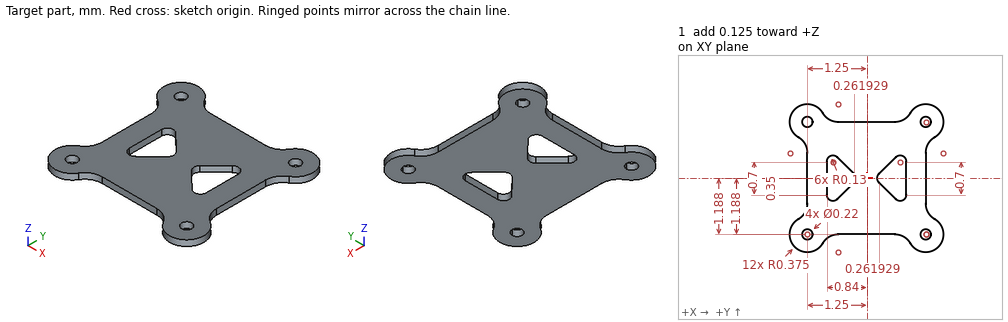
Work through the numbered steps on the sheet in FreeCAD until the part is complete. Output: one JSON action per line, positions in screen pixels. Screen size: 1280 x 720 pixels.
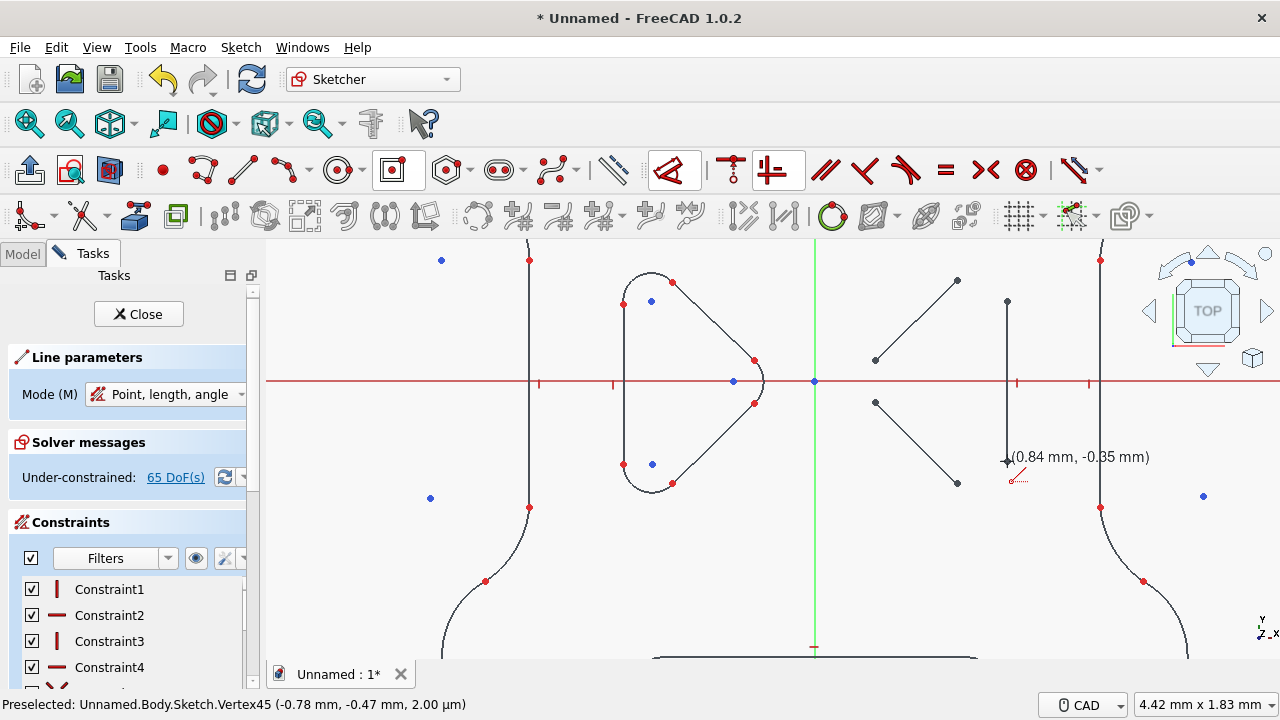
{"action": "left_click", "coordinate": [284, 170]}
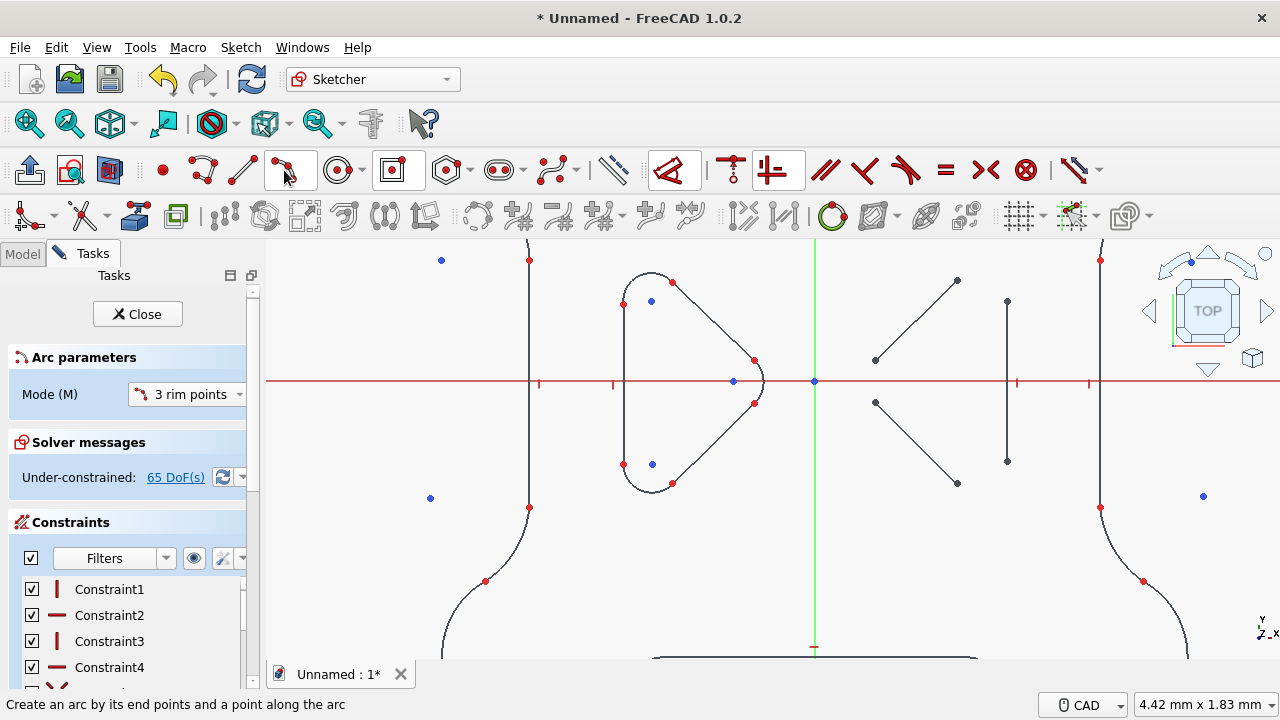
{"action": "left_click", "coordinate": [875, 403]}
{"action": "left_click", "coordinate": [875, 361]}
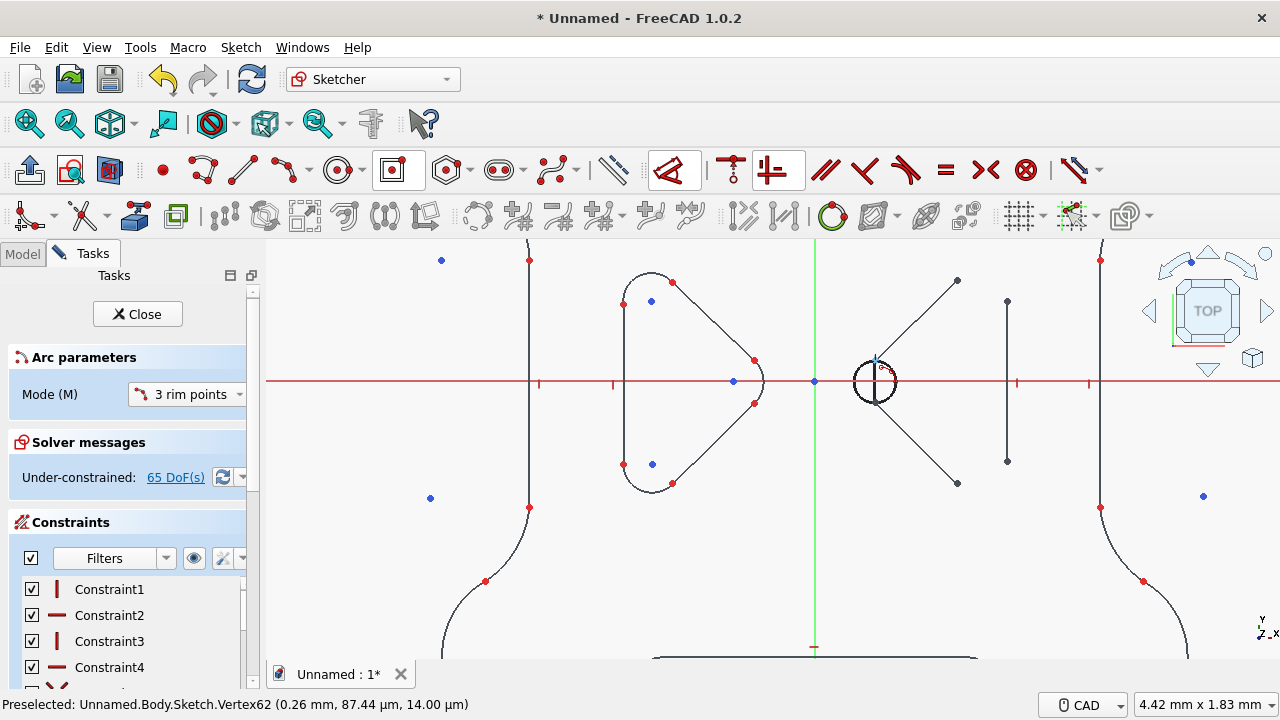
{"action": "scroll", "coordinate": [867, 372], "scroll_direction": "up", "scroll_amount": 4}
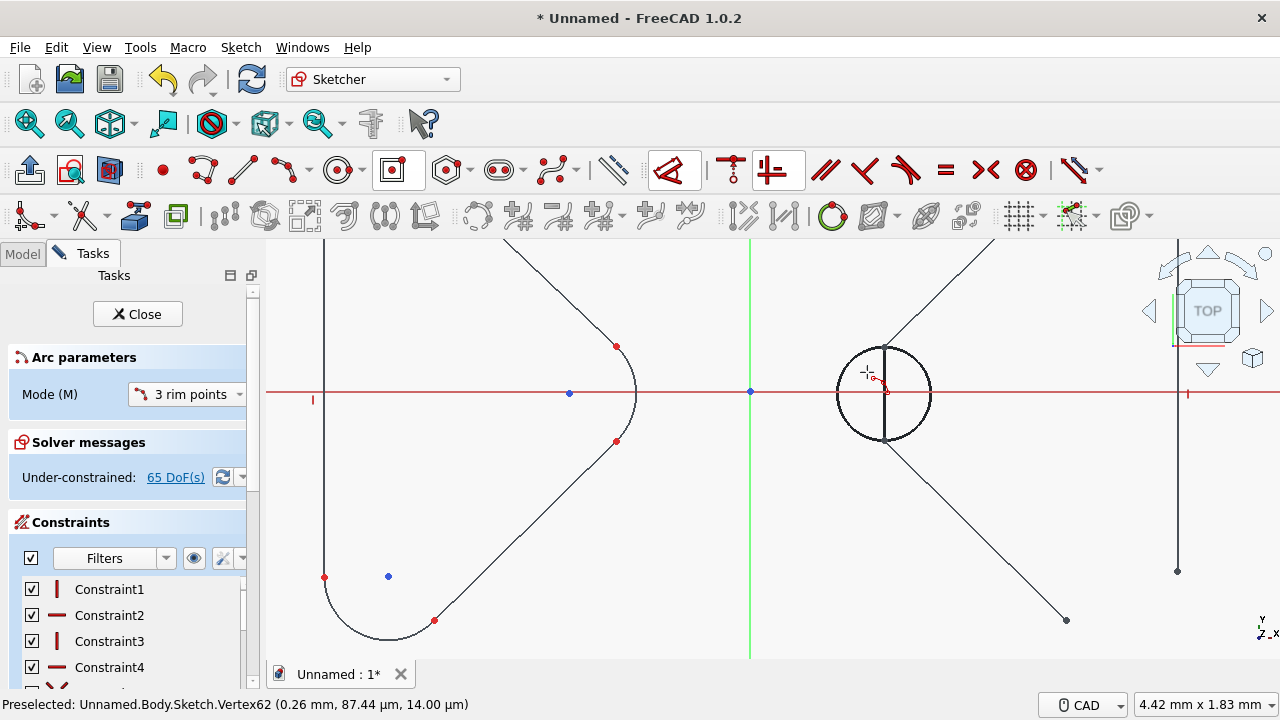
{"action": "left_click", "coordinate": [867, 371]}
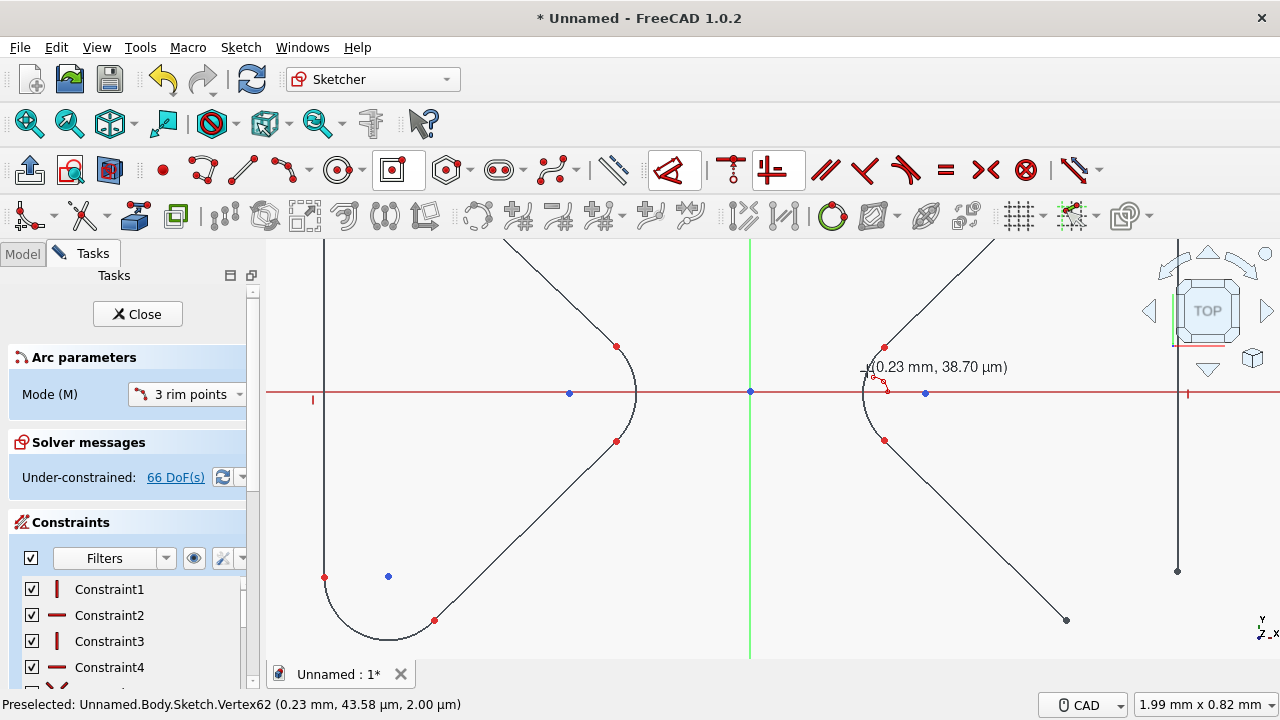
{"action": "scroll", "coordinate": [695, 460], "scroll_direction": "down", "scroll_amount": 9}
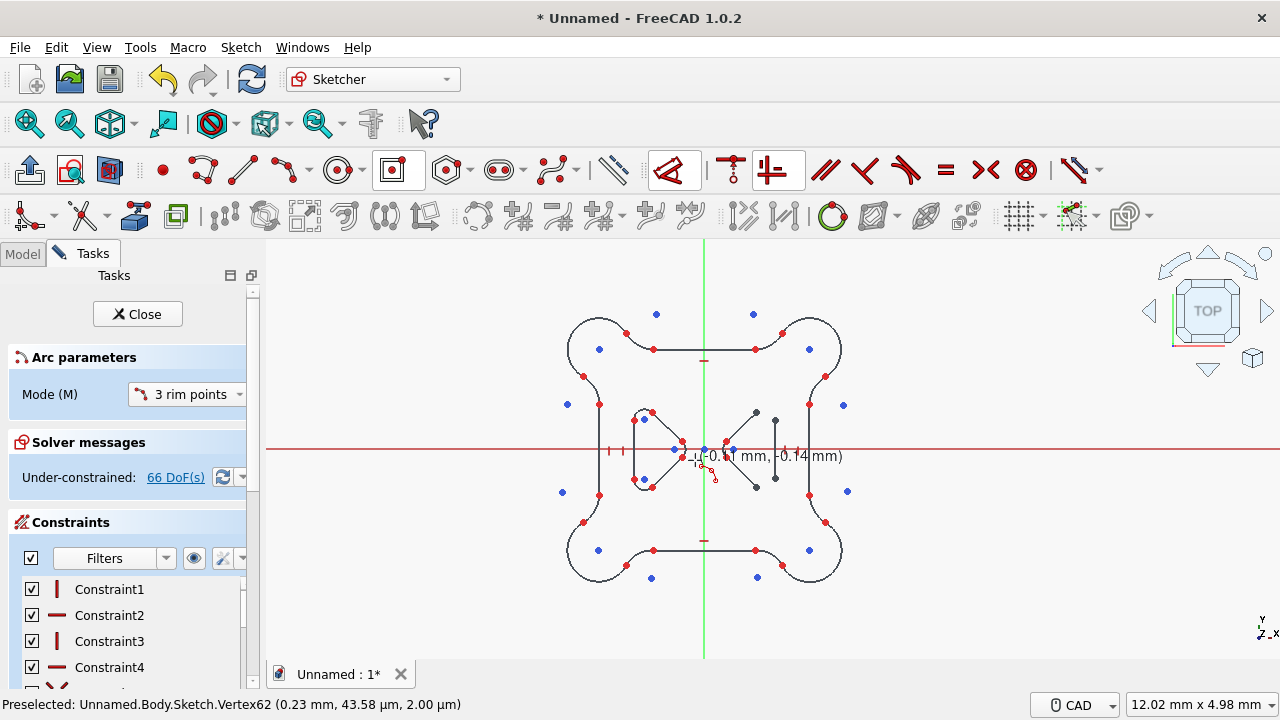
{"action": "left_click", "coordinate": [757, 412]}
{"action": "left_click", "coordinate": [775, 420]}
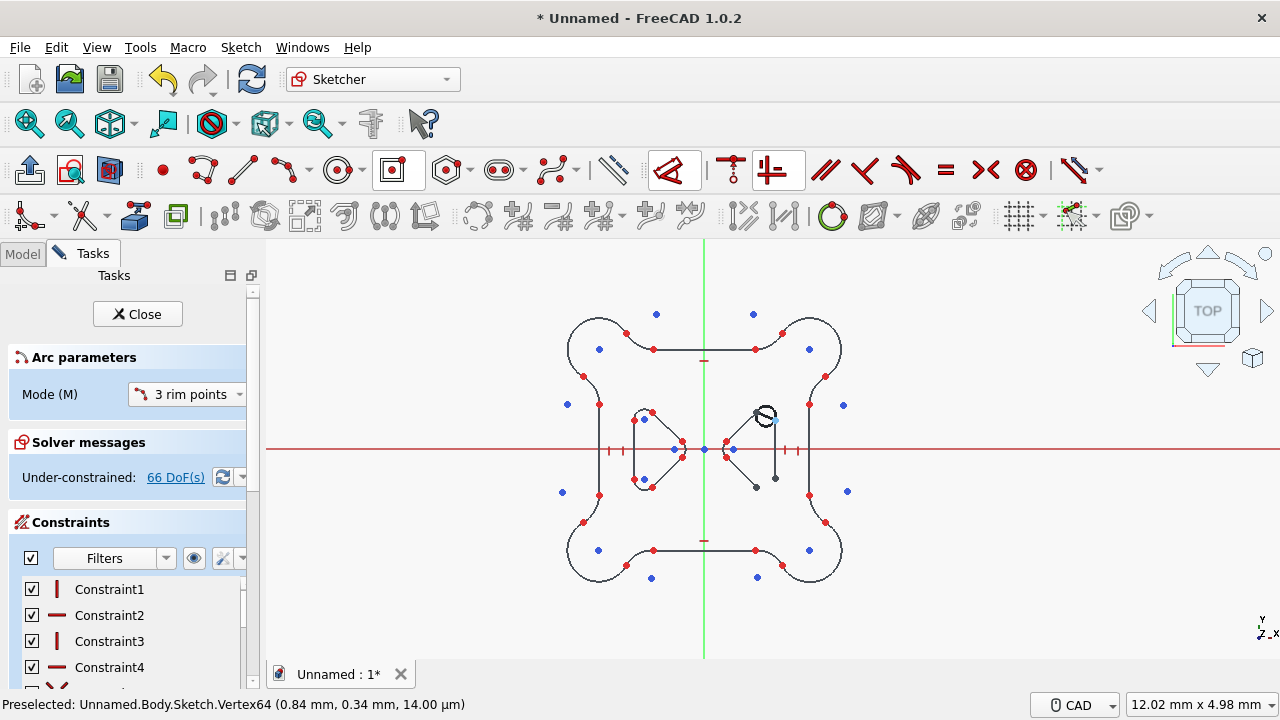
{"action": "scroll", "coordinate": [769, 410], "scroll_direction": "up", "scroll_amount": 5}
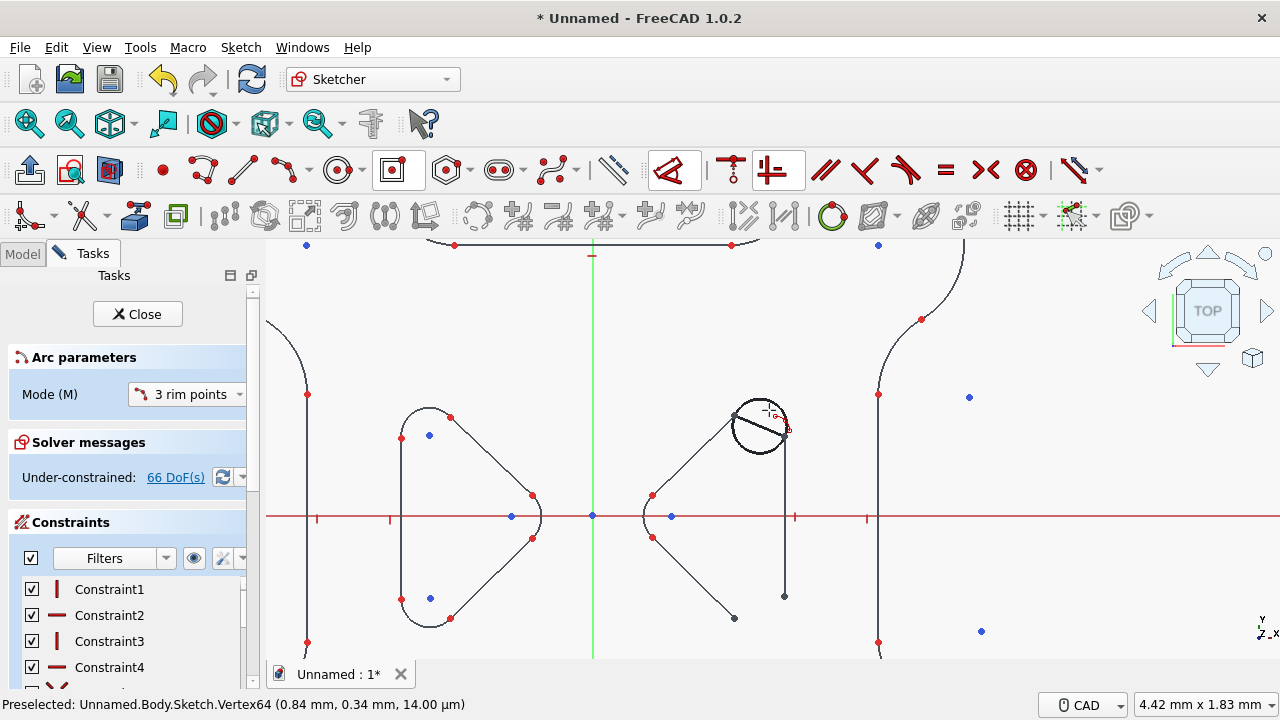
{"action": "left_click", "coordinate": [767, 408]}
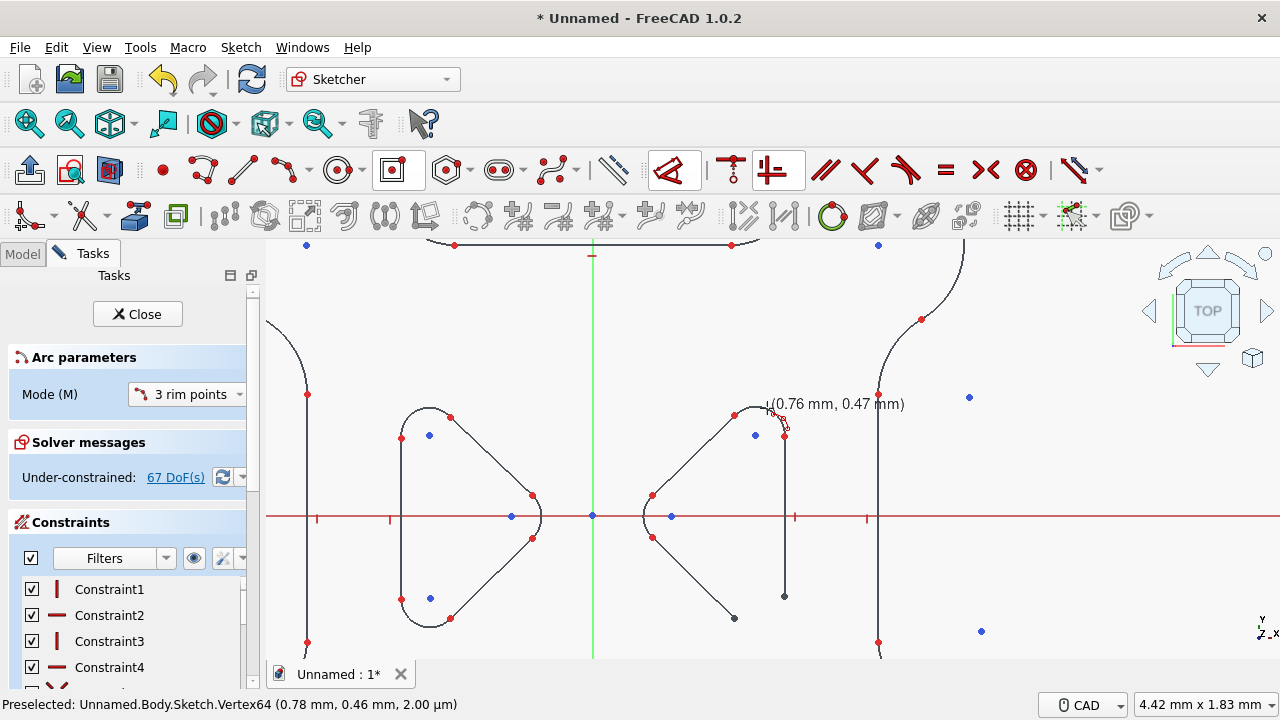
{"action": "left_click", "coordinate": [785, 597]}
{"action": "left_click", "coordinate": [735, 619]}
{"action": "left_click", "coordinate": [767, 623]}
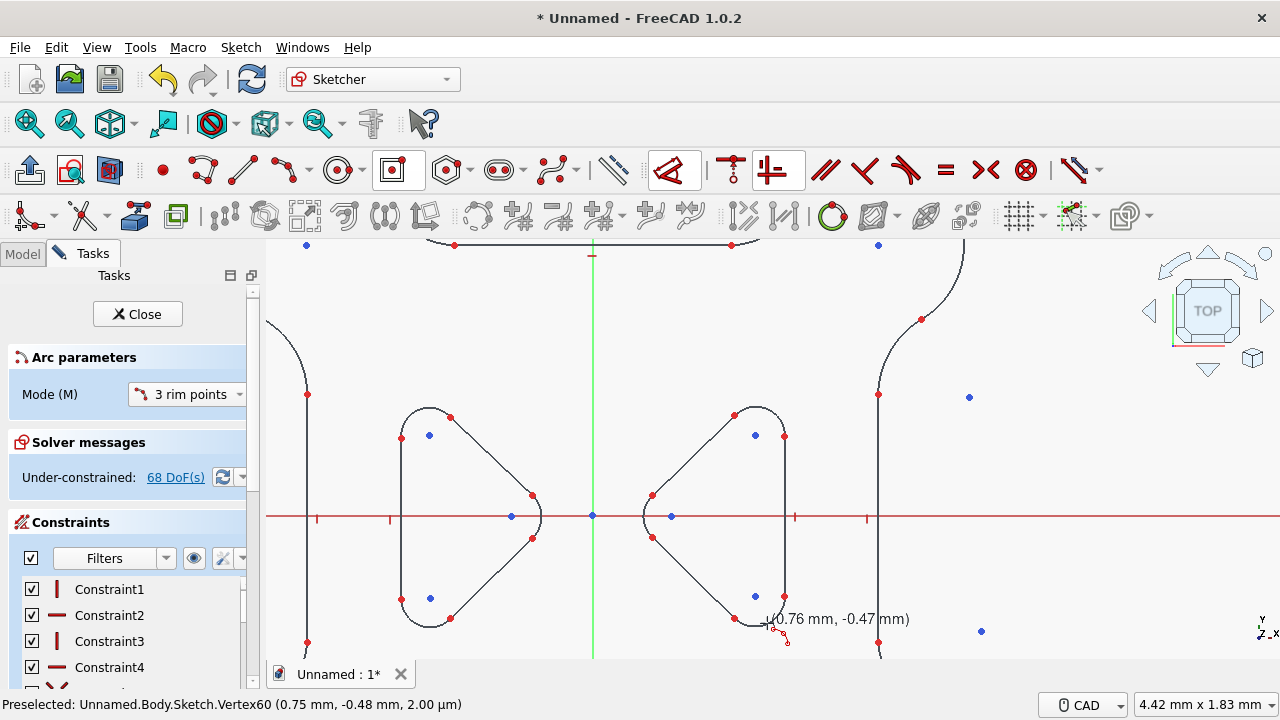
{"action": "left_click", "coordinate": [338, 170]}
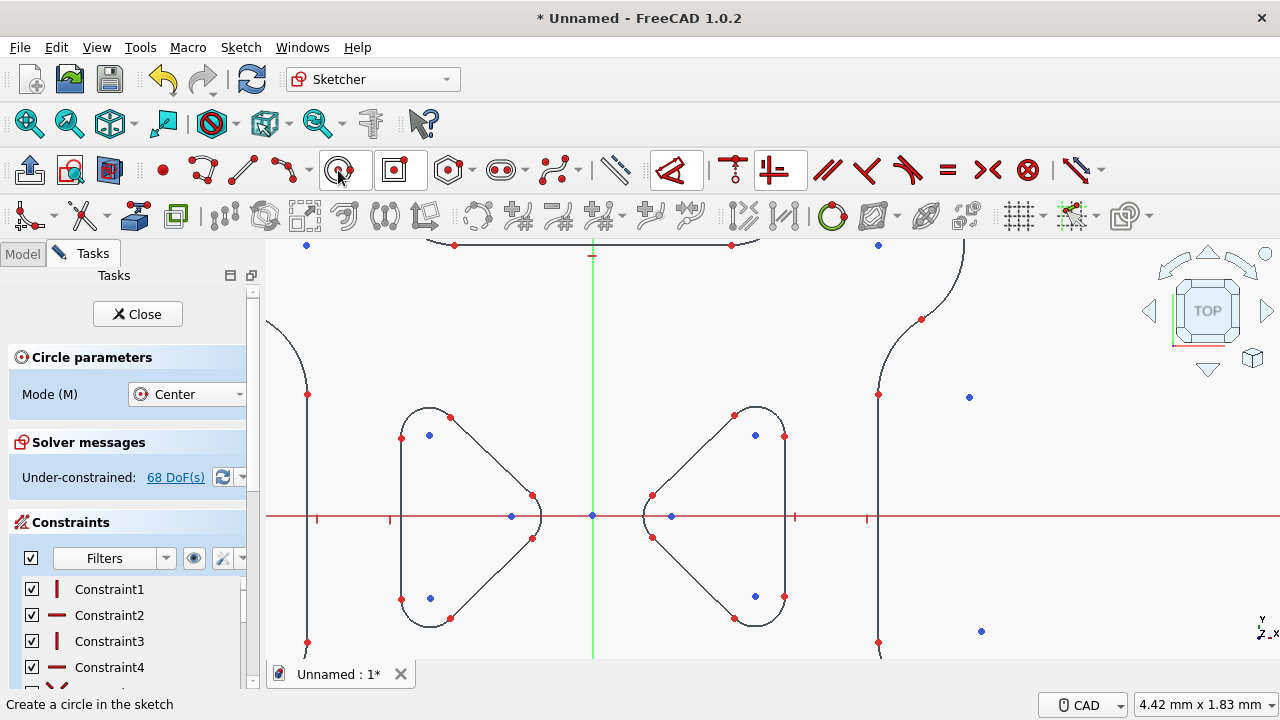
{"action": "scroll", "coordinate": [770, 410], "scroll_direction": "down", "scroll_amount": 5}